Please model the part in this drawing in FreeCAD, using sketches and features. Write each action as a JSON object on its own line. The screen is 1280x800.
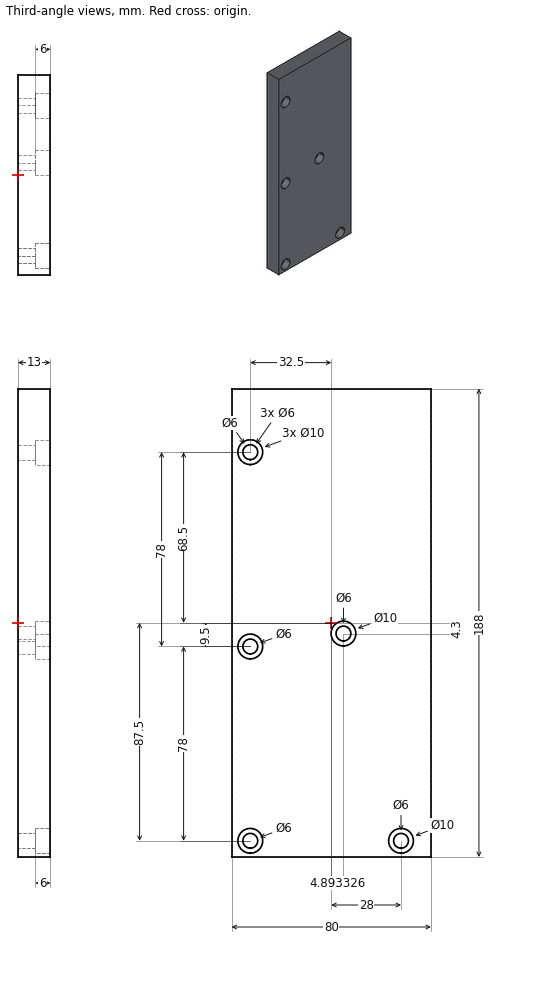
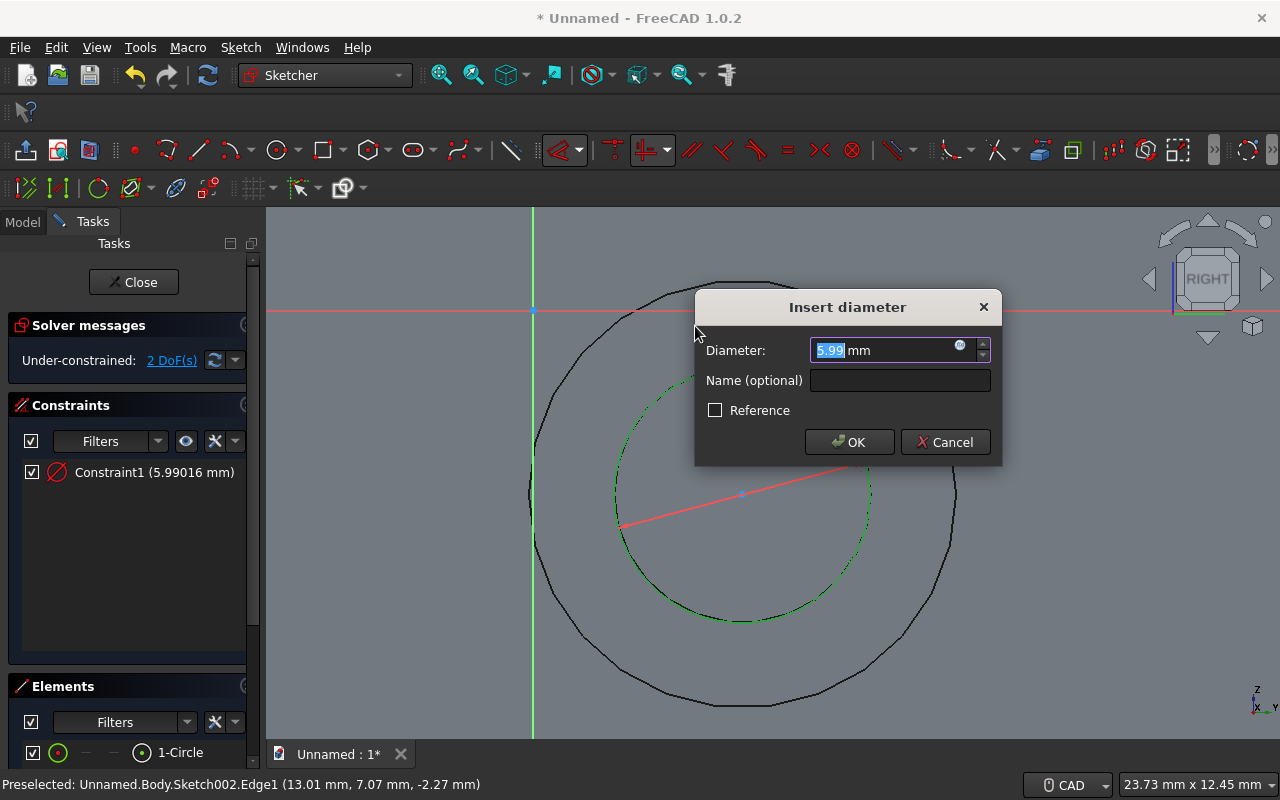
{"action": "type", "text": "6"}
{"action": "key", "text": "Return"}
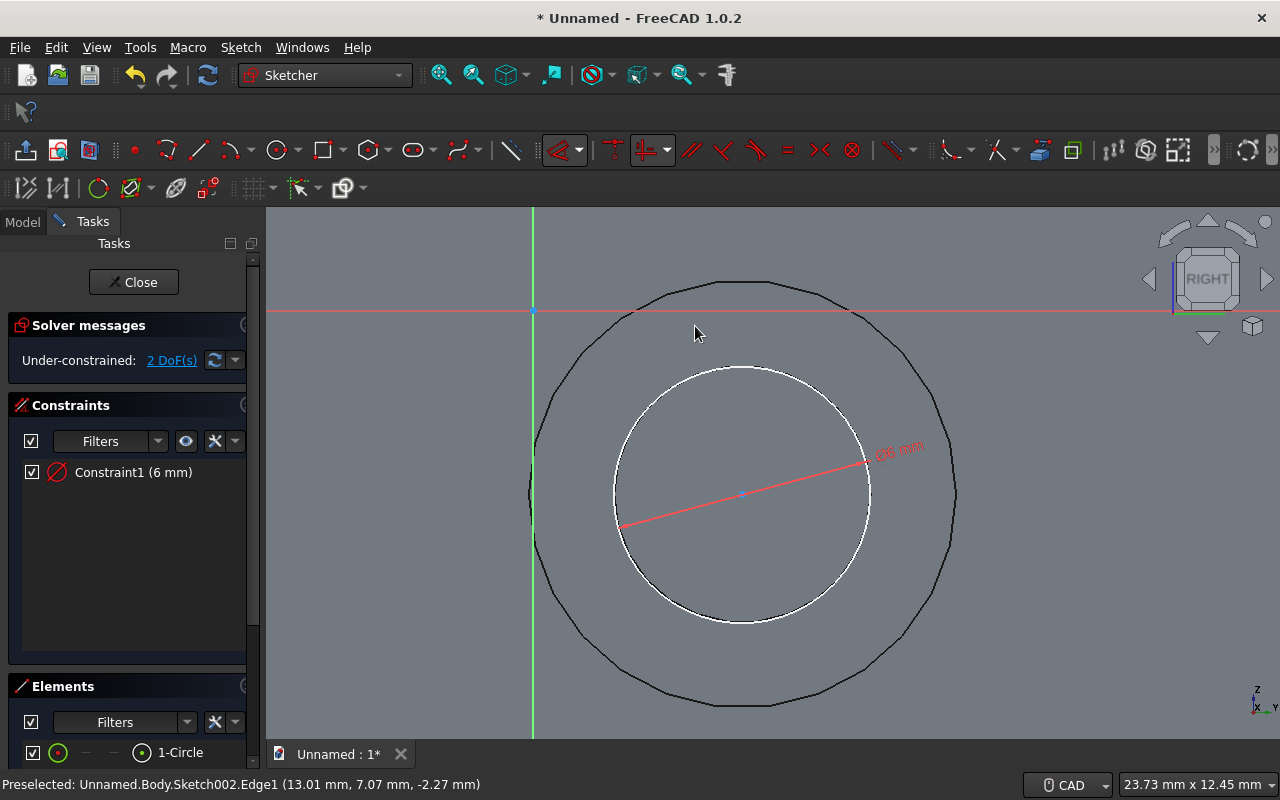
{"action": "left_click", "coordinate": [742, 495]}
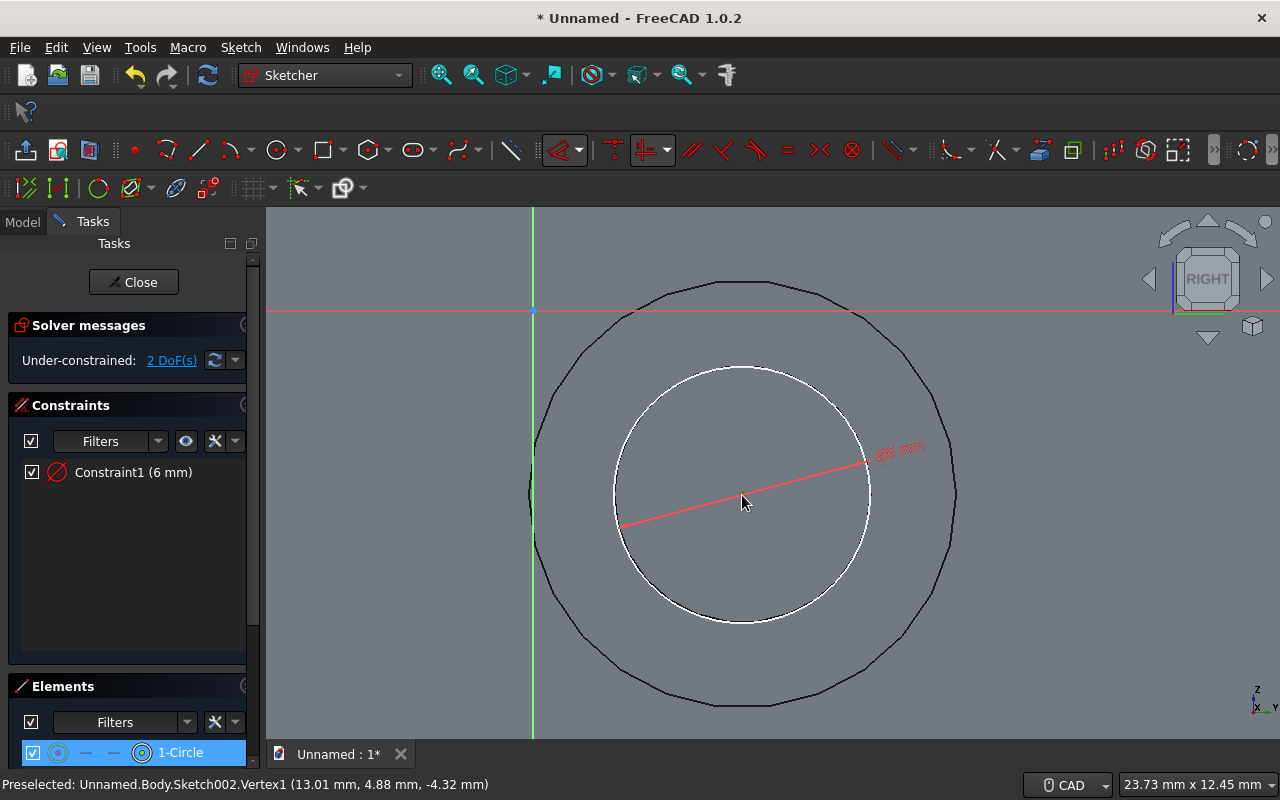
{"action": "key", "text": "i"}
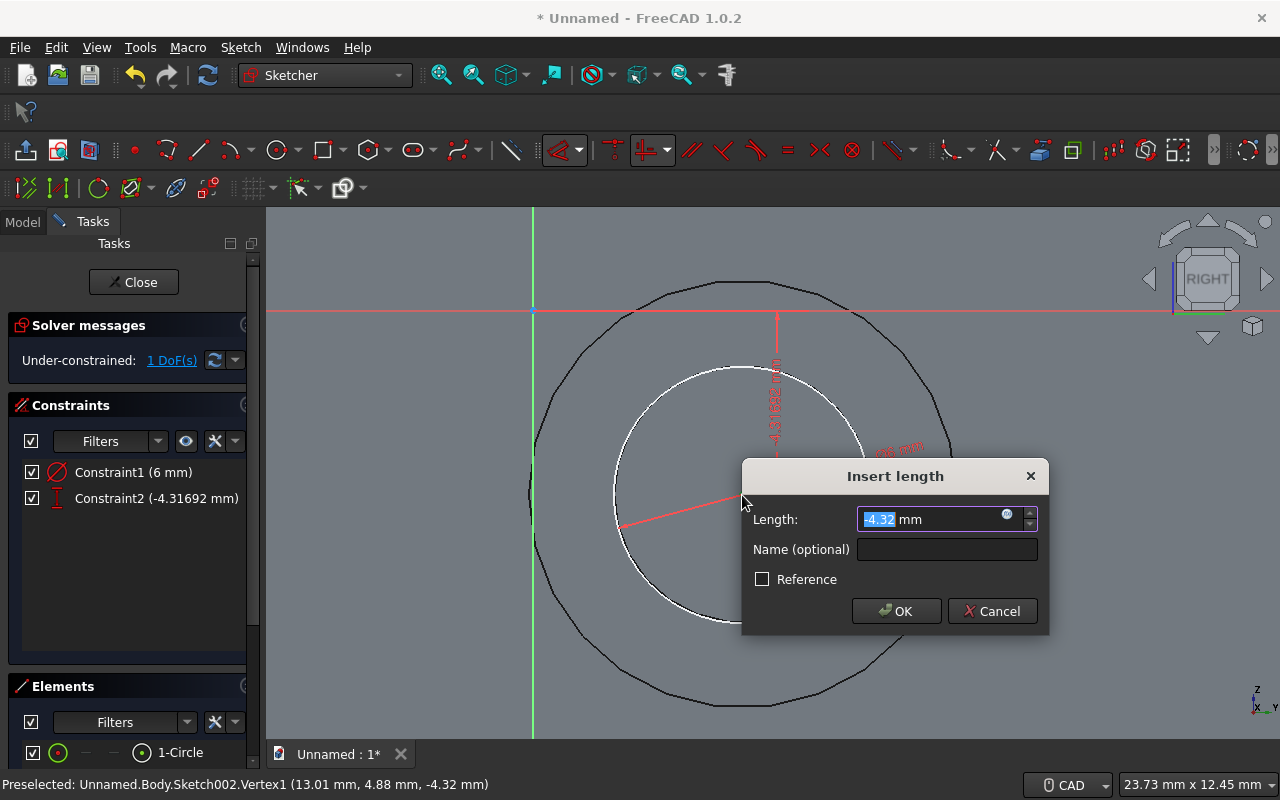
{"action": "type", "text": "-4.3"}
{"action": "key", "text": "Return"}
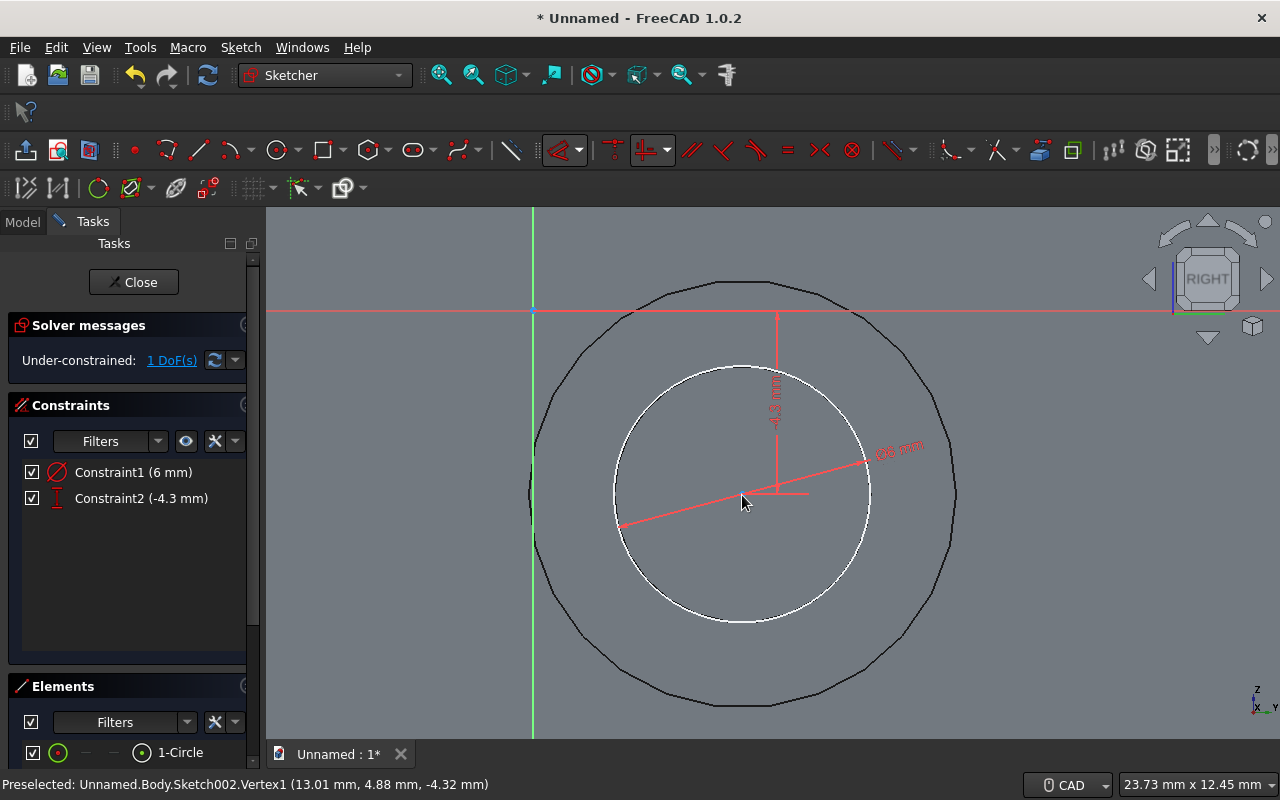
{"action": "left_click", "coordinate": [742, 494]}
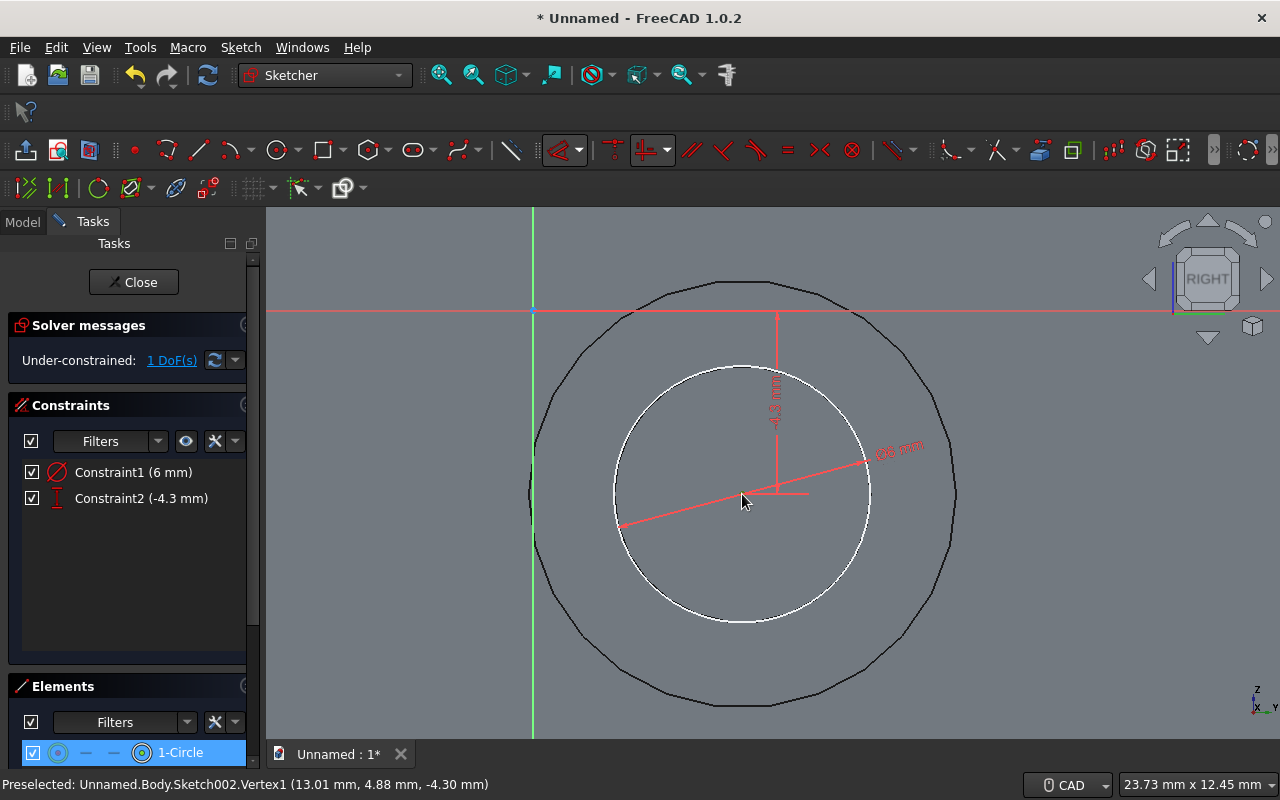
{"action": "key", "text": "l"}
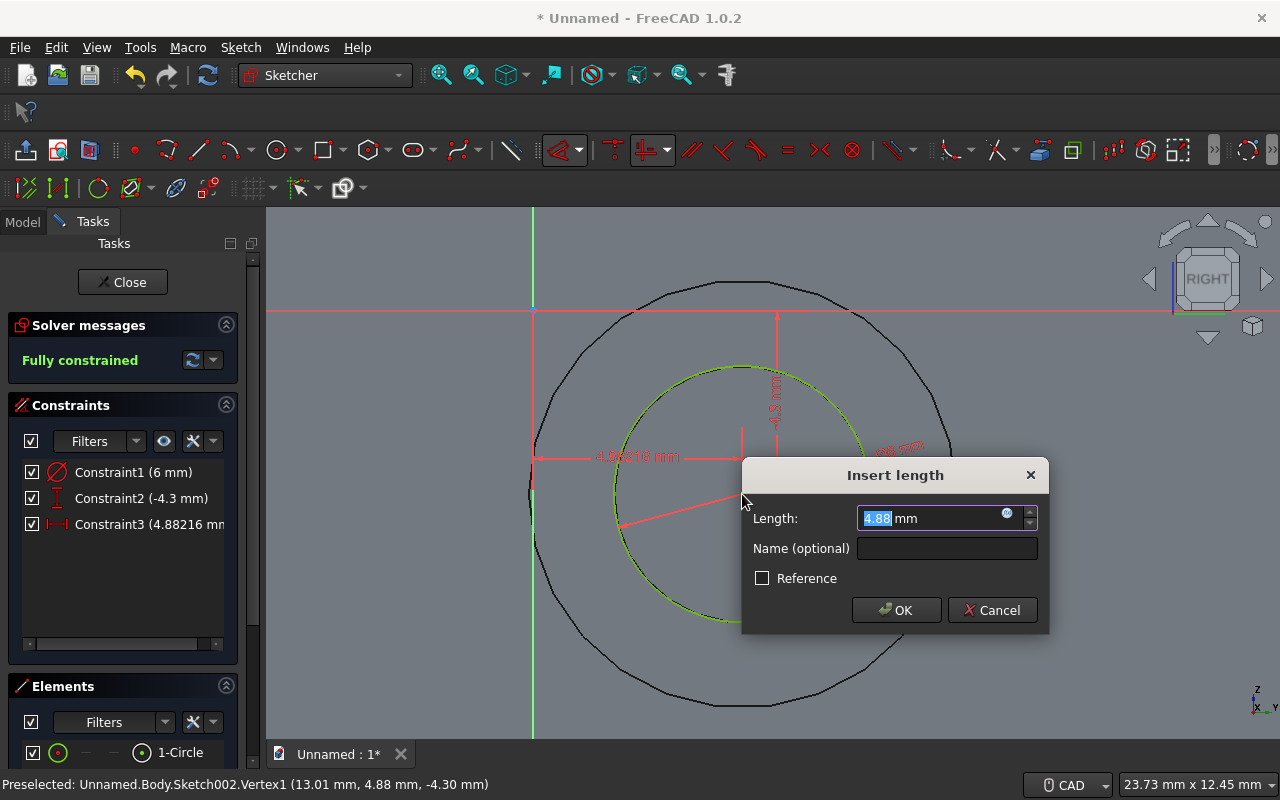
{"action": "type", "text": "4.893326"}
{"action": "key", "text": "Return"}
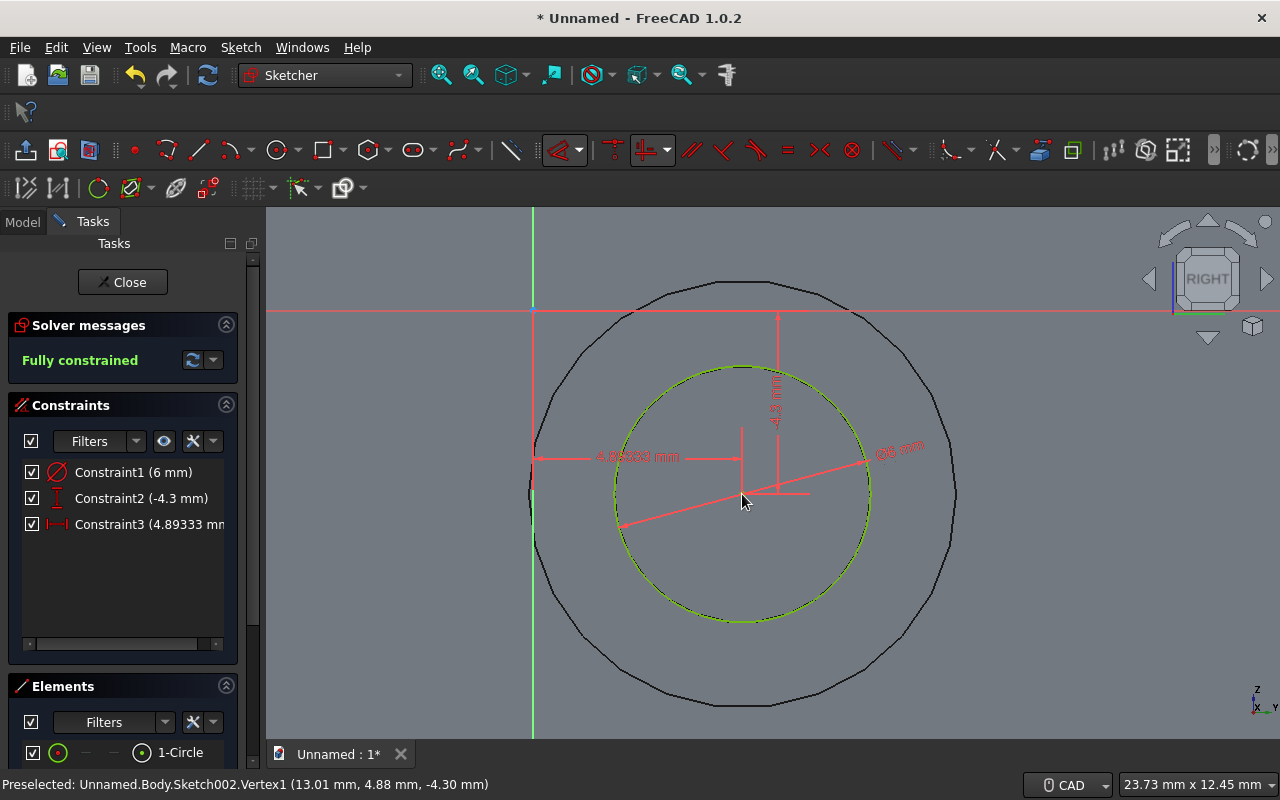
{"action": "left_click", "coordinate": [123, 282]}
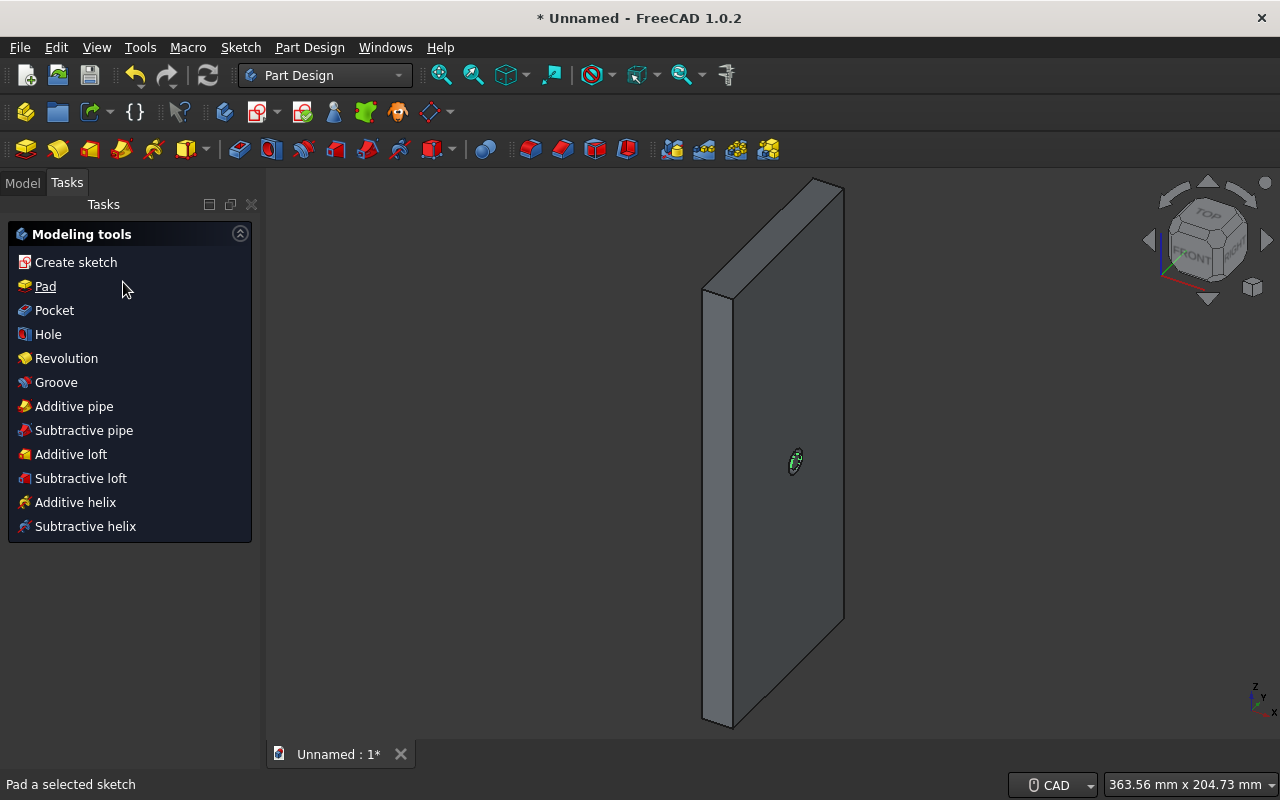
{"action": "left_click", "coordinate": [240, 150]}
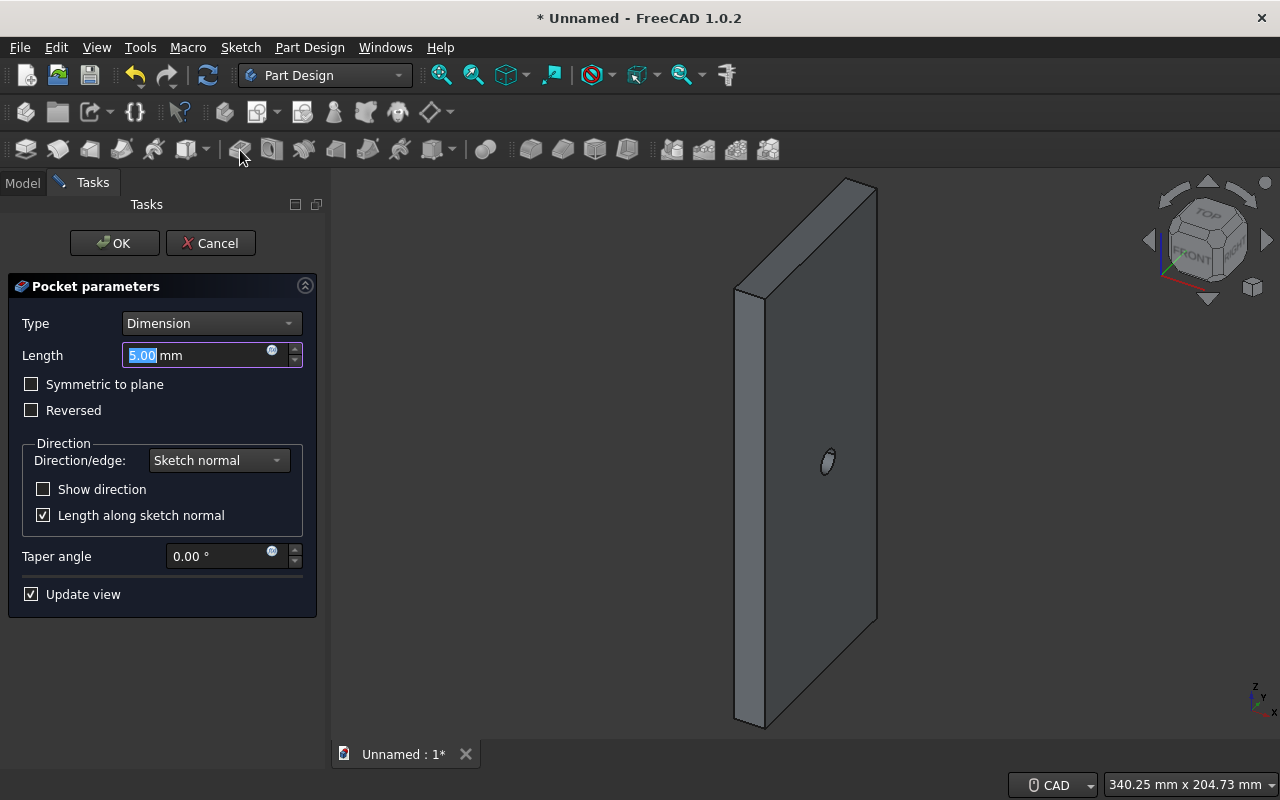
{"action": "left_click", "coordinate": [212, 324]}